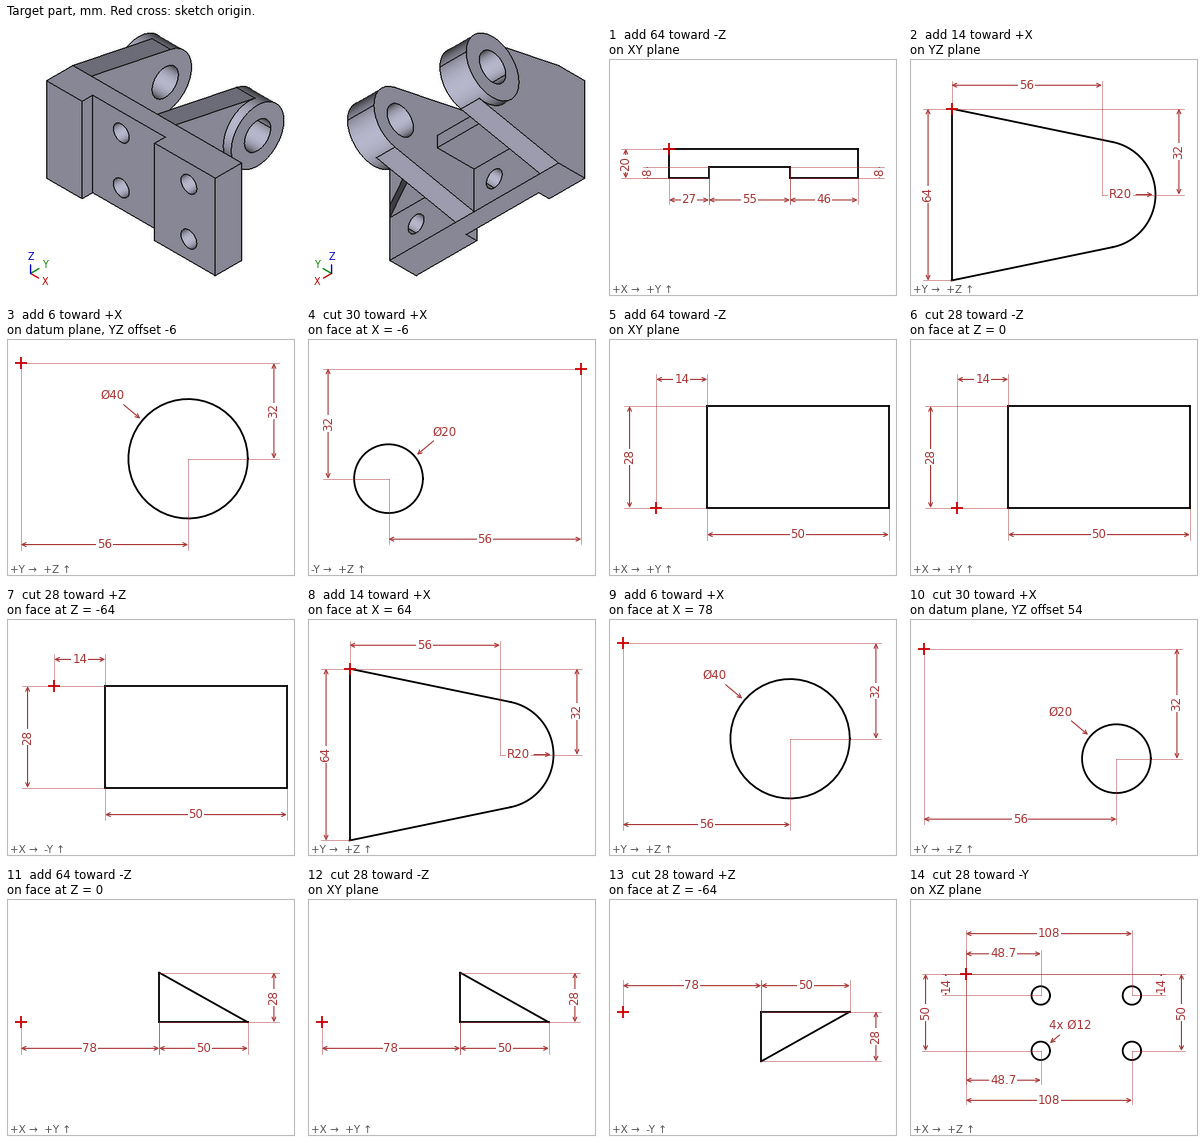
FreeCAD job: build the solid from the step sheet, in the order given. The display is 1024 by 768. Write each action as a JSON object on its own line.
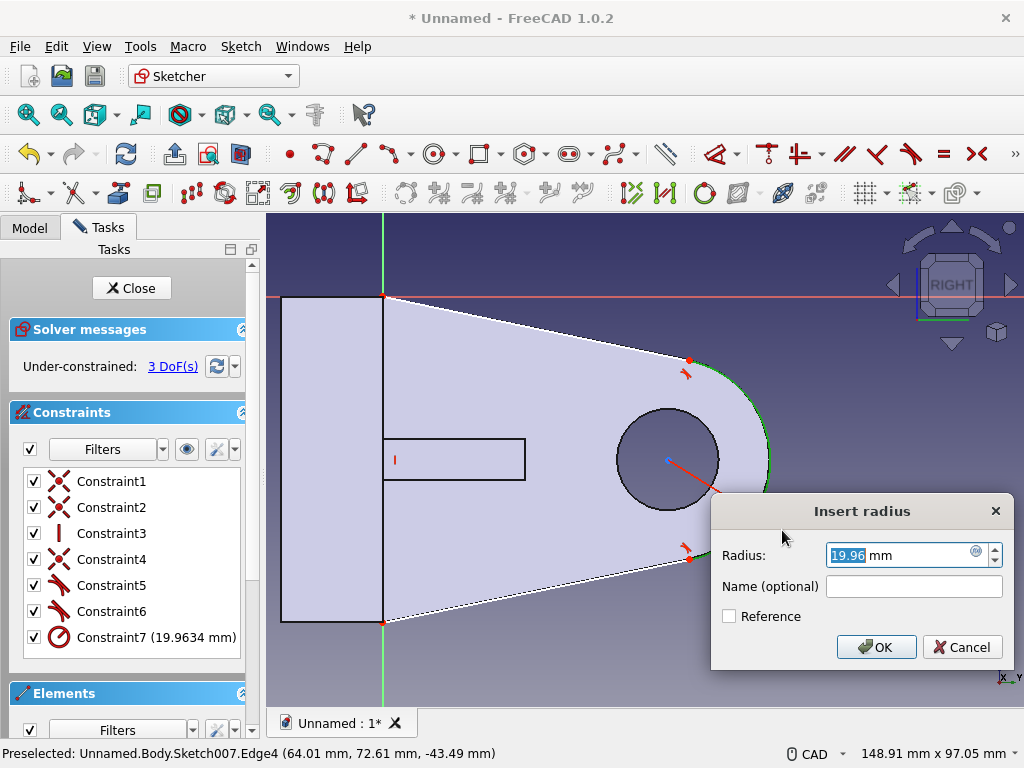
{"action": "type", "text": "20"}
{"action": "key", "text": "Return"}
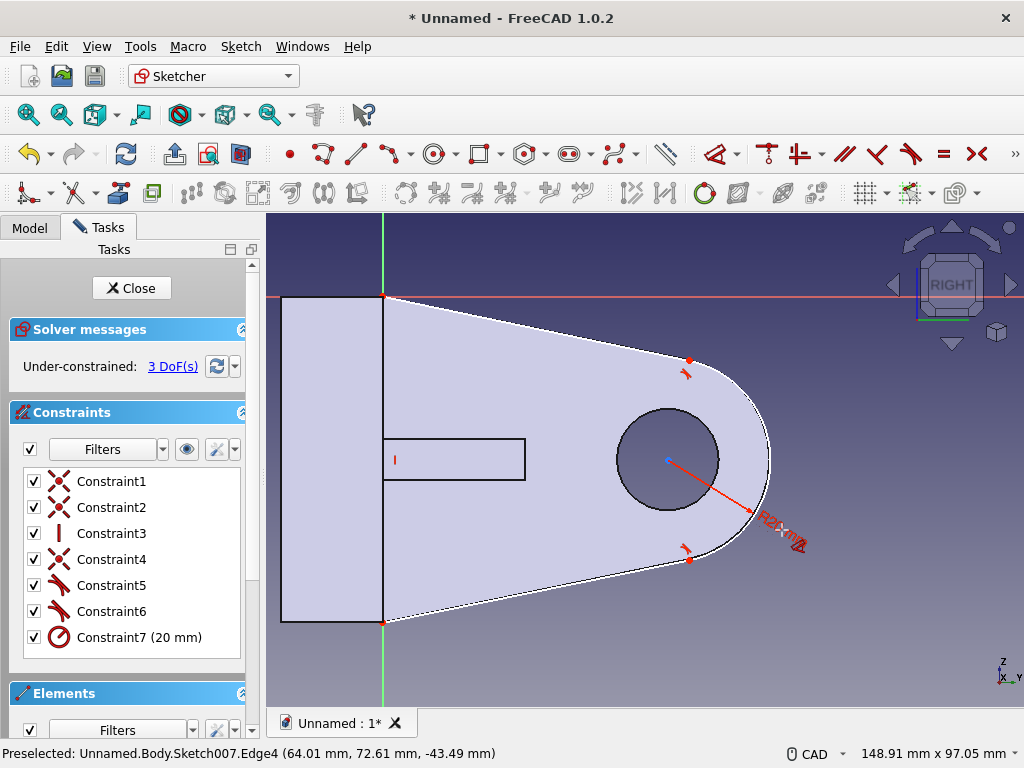
{"action": "left_click", "coordinate": [383, 395]}
{"action": "left_click", "coordinate": [349, 460]}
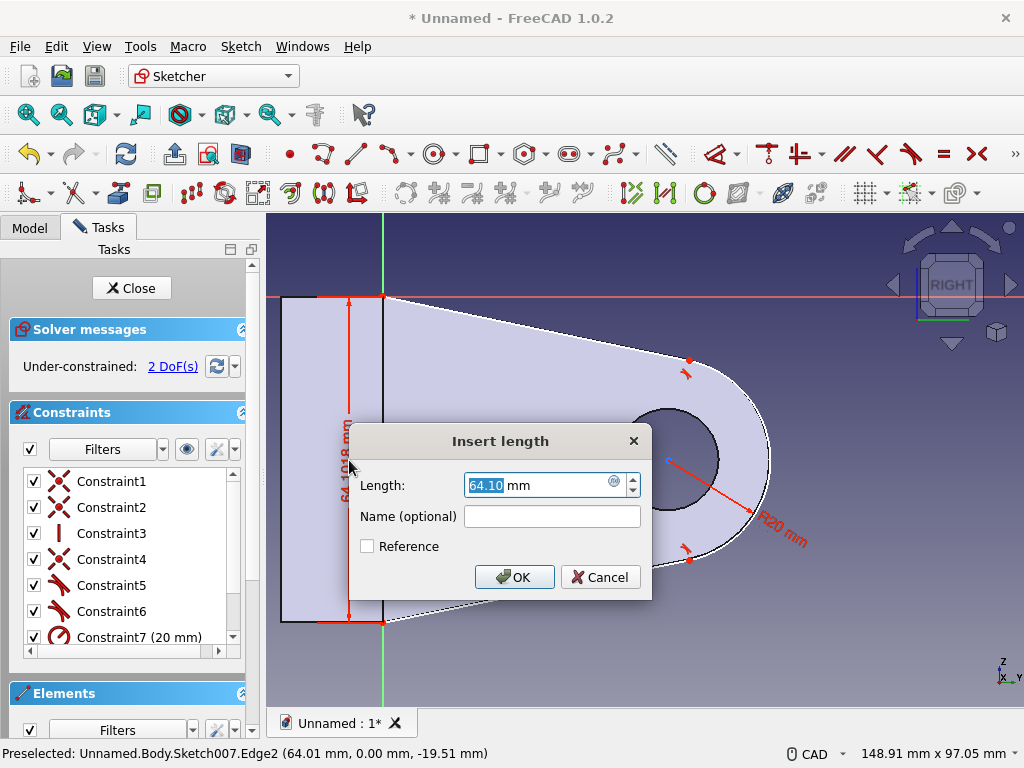
{"action": "type", "text": "64"}
{"action": "key", "text": "Return"}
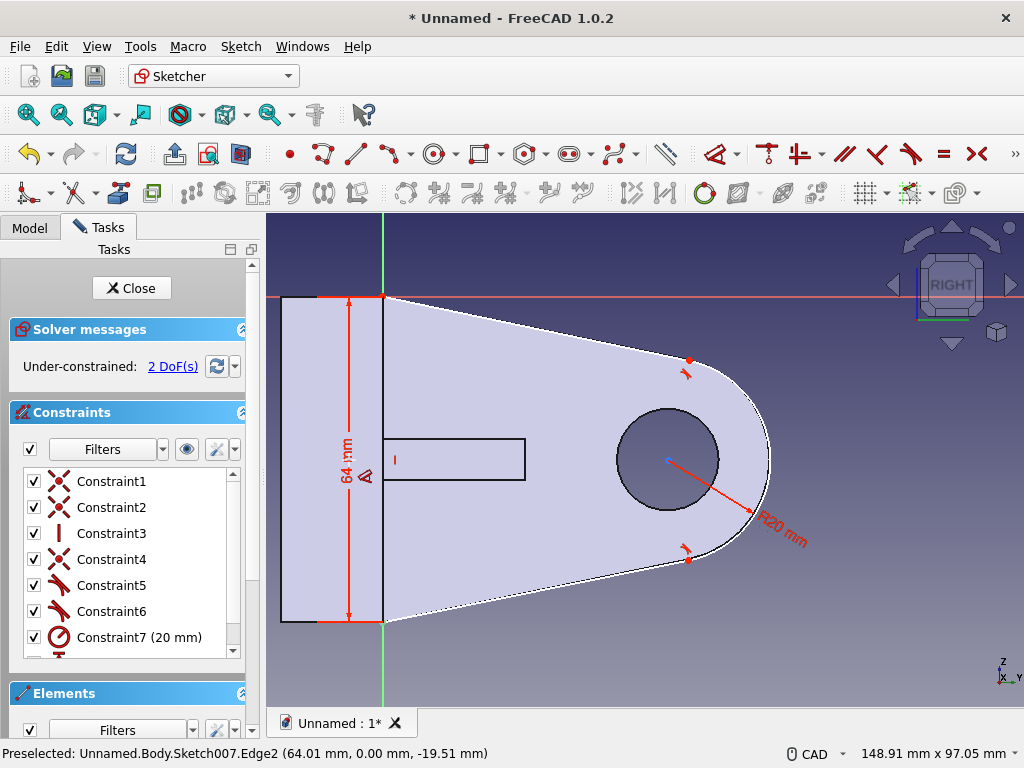
{"action": "left_click", "coordinate": [669, 461]}
{"action": "left_click", "coordinate": [526, 263]}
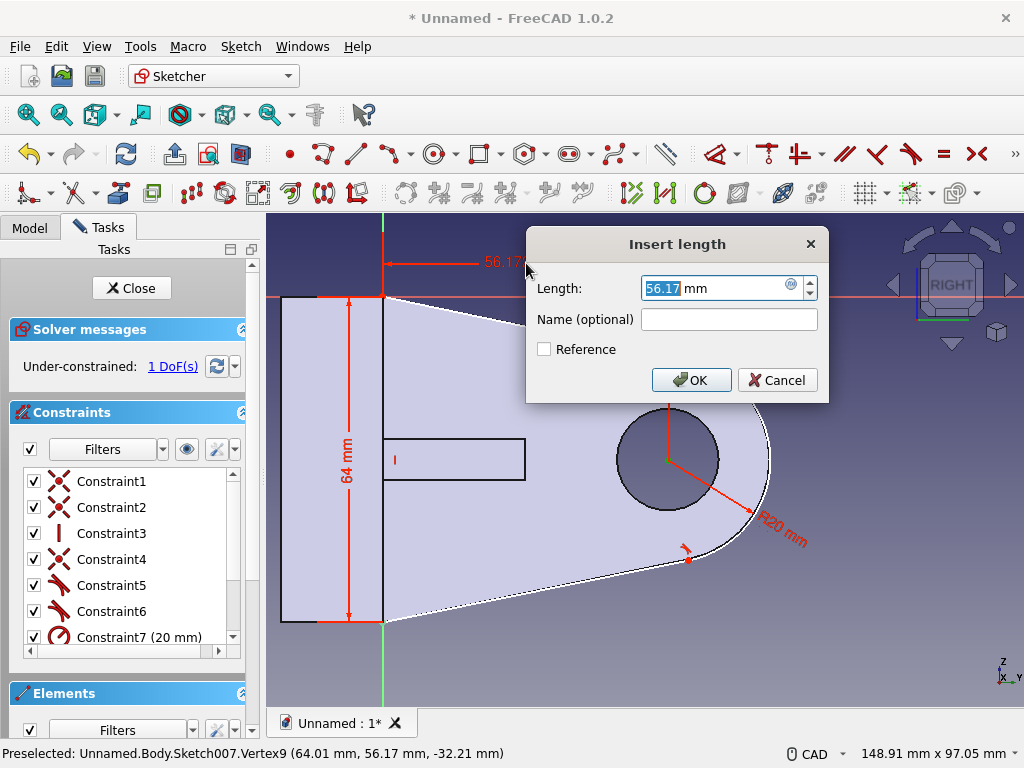
{"action": "type", "text": "56"}
{"action": "key", "text": "Return"}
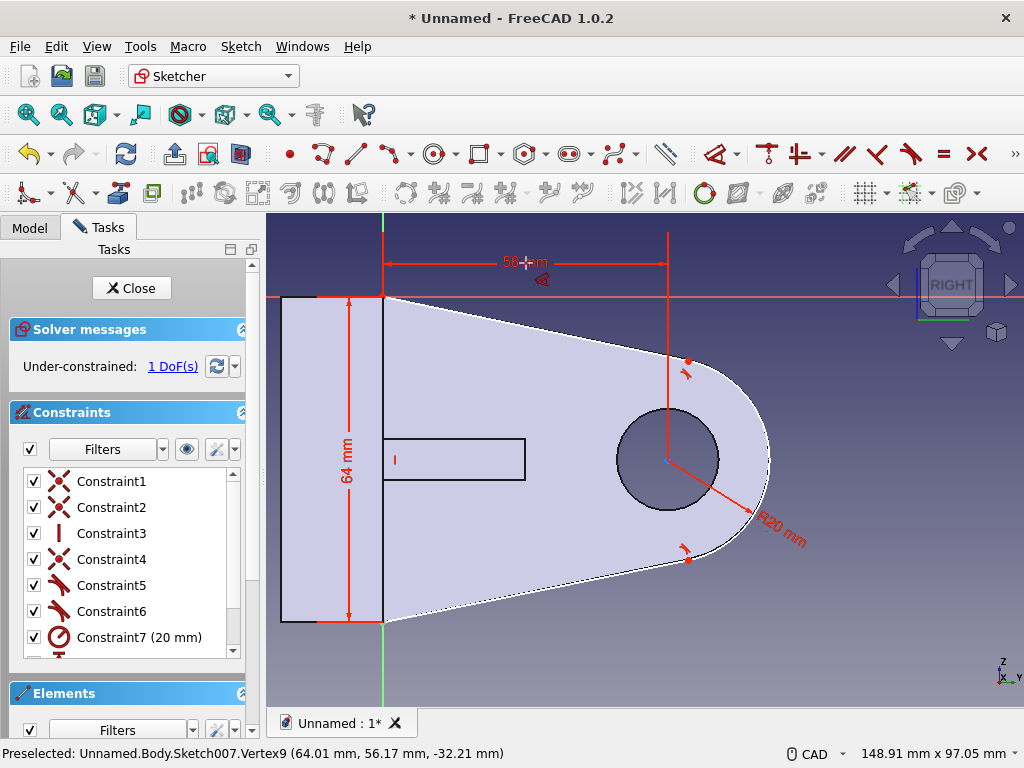
{"action": "left_click", "coordinate": [668, 461]}
{"action": "left_click", "coordinate": [349, 379]}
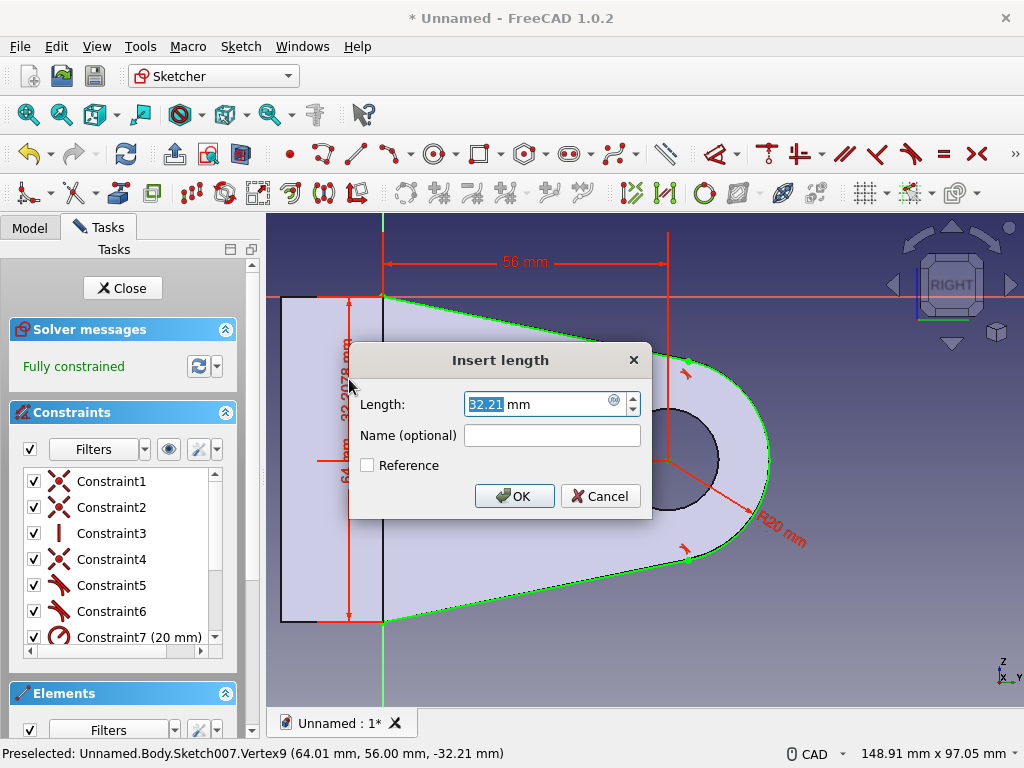
{"action": "type", "text": "32"}
{"action": "key", "text": "Return"}
{"action": "key", "text": "Escape"}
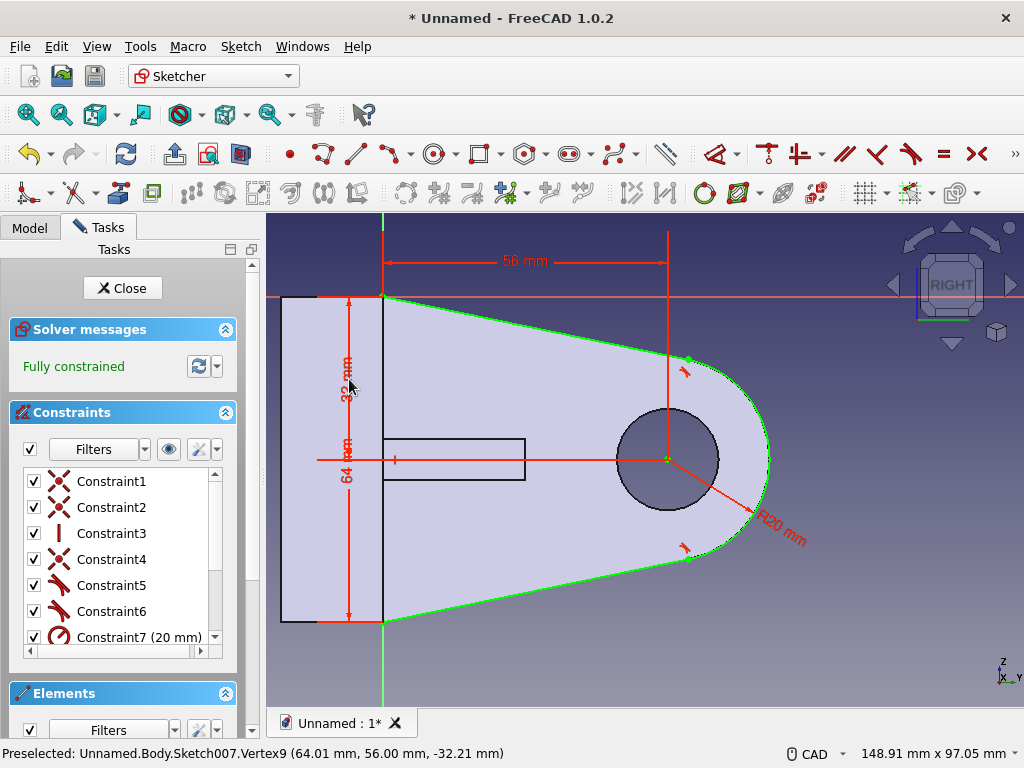
{"action": "left_click", "coordinate": [123, 288]}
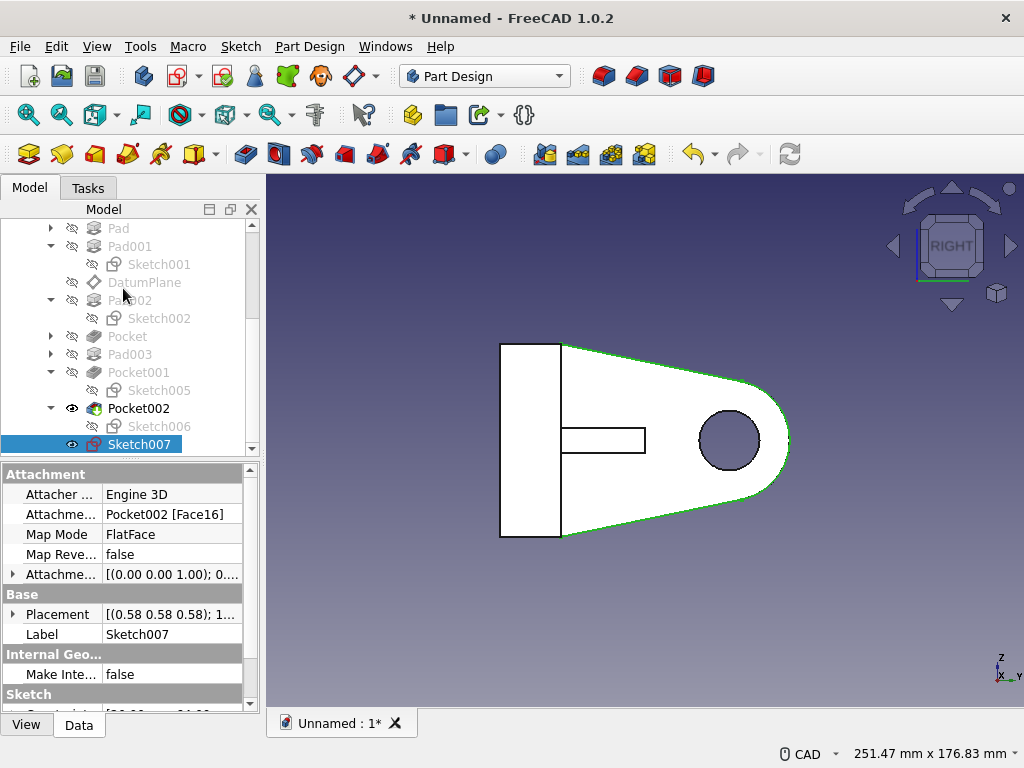
{"action": "left_click", "coordinate": [29, 154]}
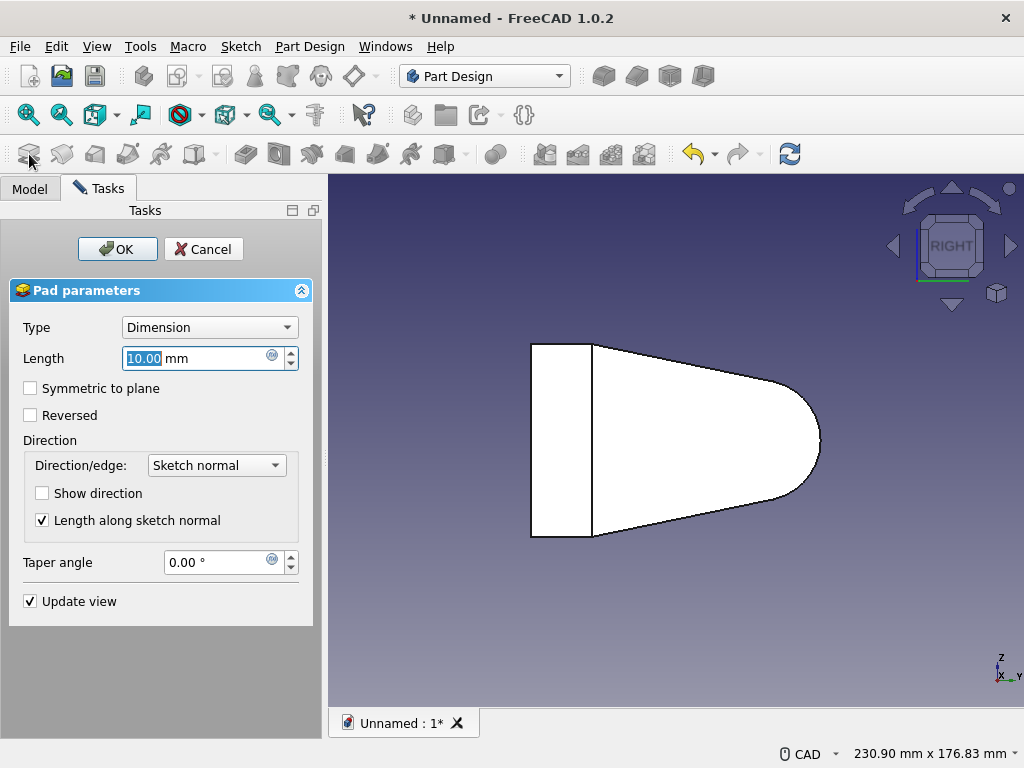
{"action": "type", "text": "14"}
{"action": "key", "text": "Tab"}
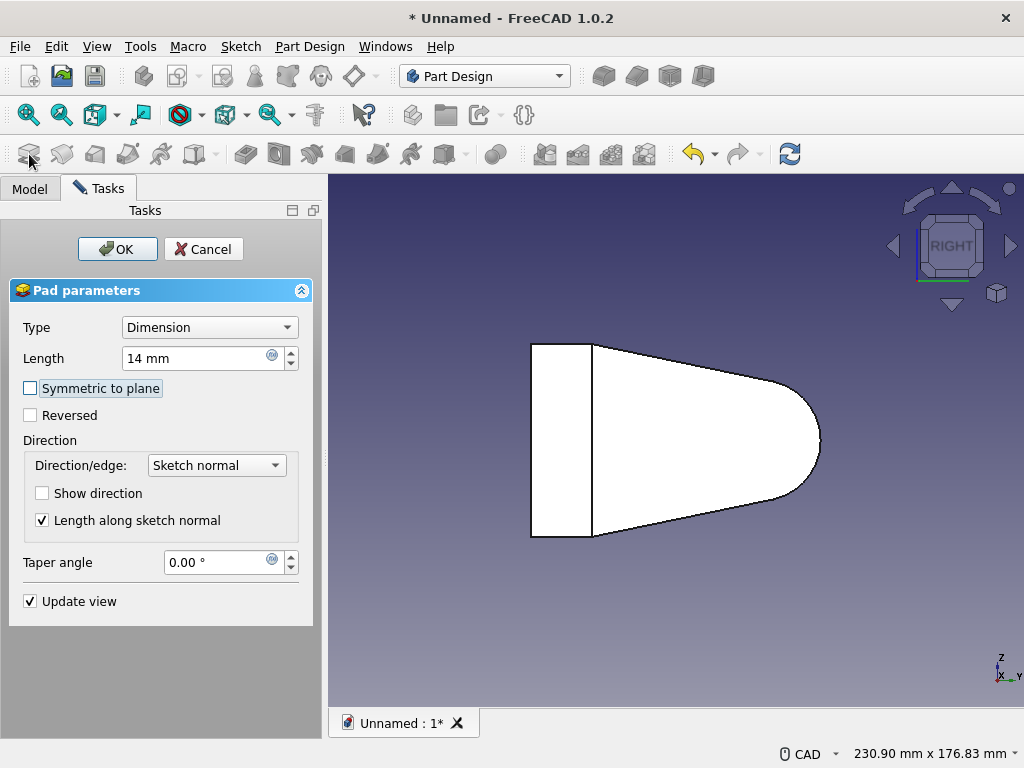
{"action": "left_click", "coordinate": [118, 249]}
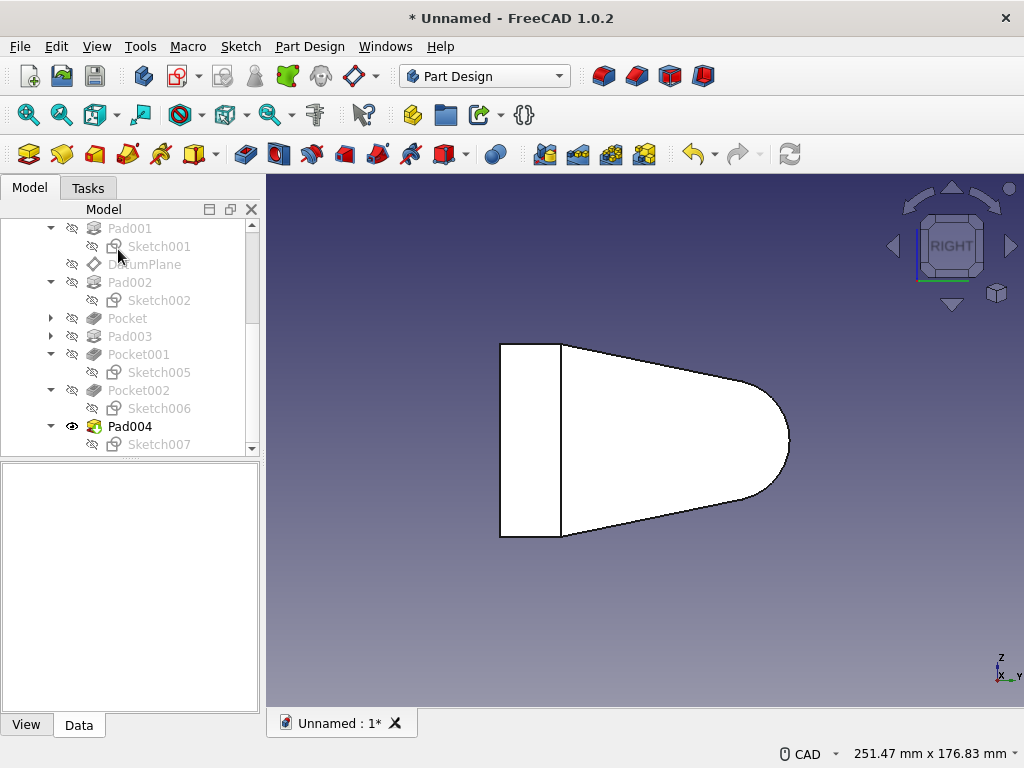
{"action": "left_click", "coordinate": [29, 116]}